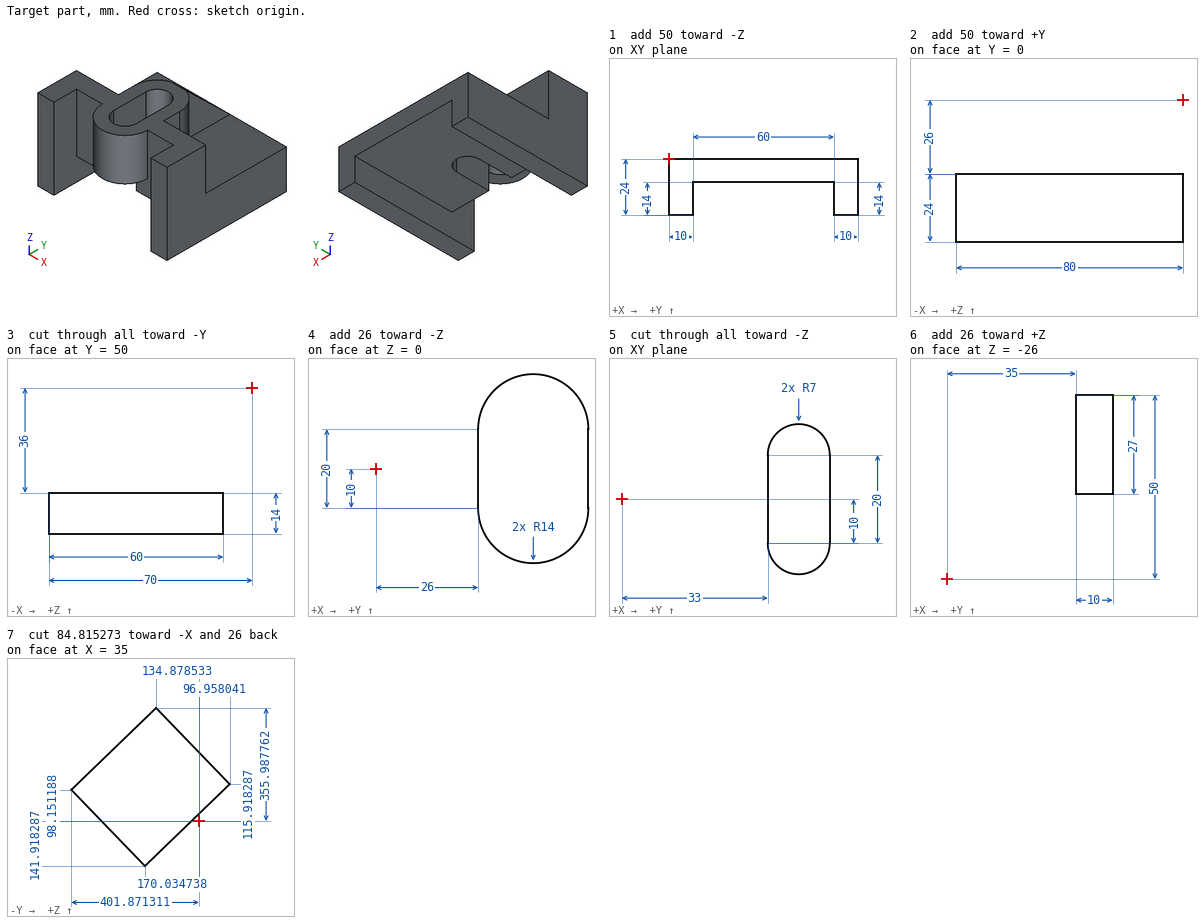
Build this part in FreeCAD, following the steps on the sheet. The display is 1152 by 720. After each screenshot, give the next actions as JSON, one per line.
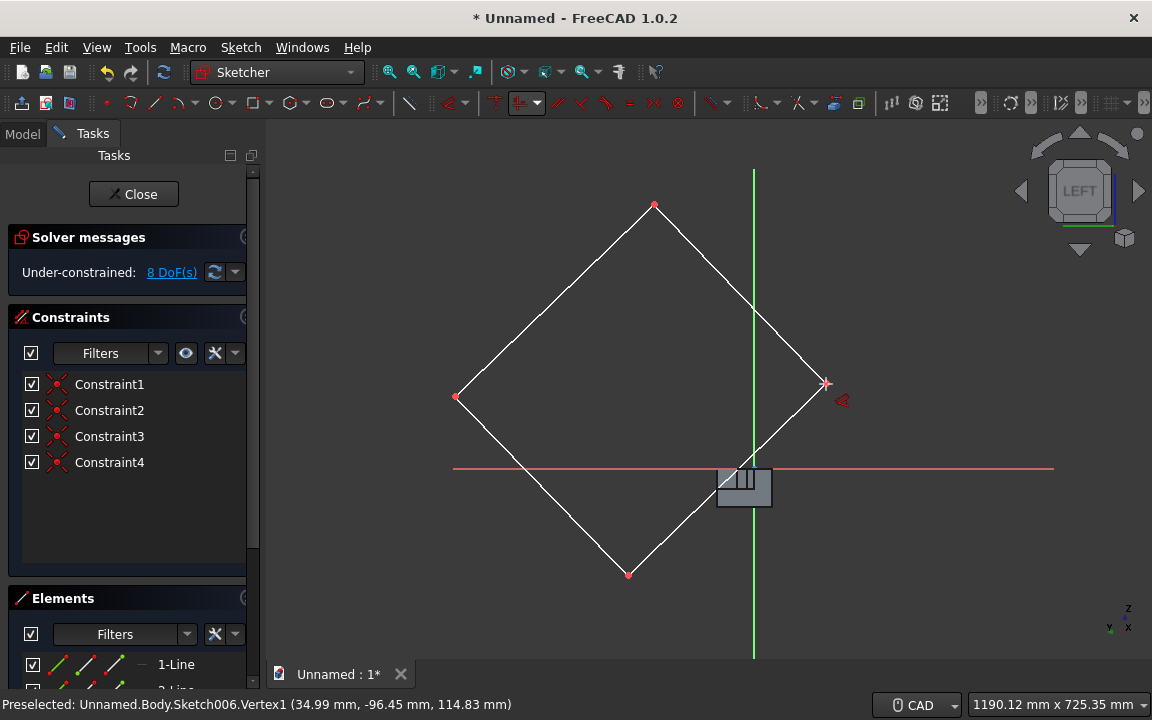
{"action": "left_click", "coordinate": [826, 384]}
{"action": "left_click", "coordinate": [790, 503]}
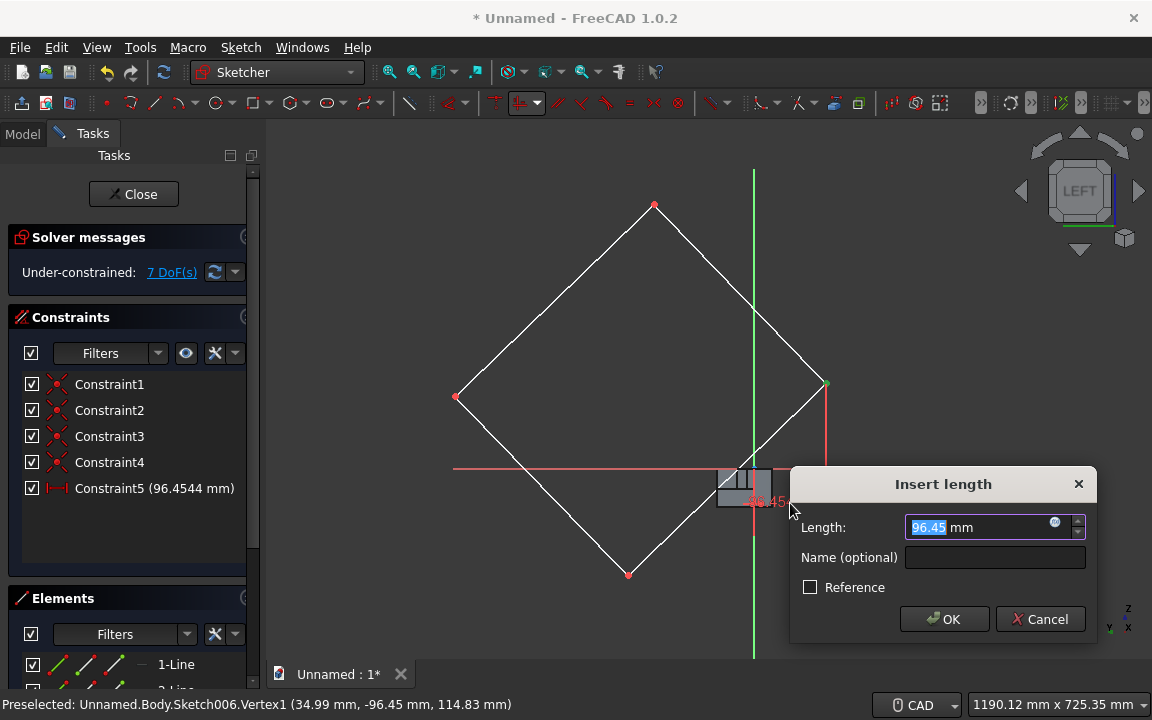
{"action": "type", "text": "96.958041"}
{"action": "key", "text": "Return"}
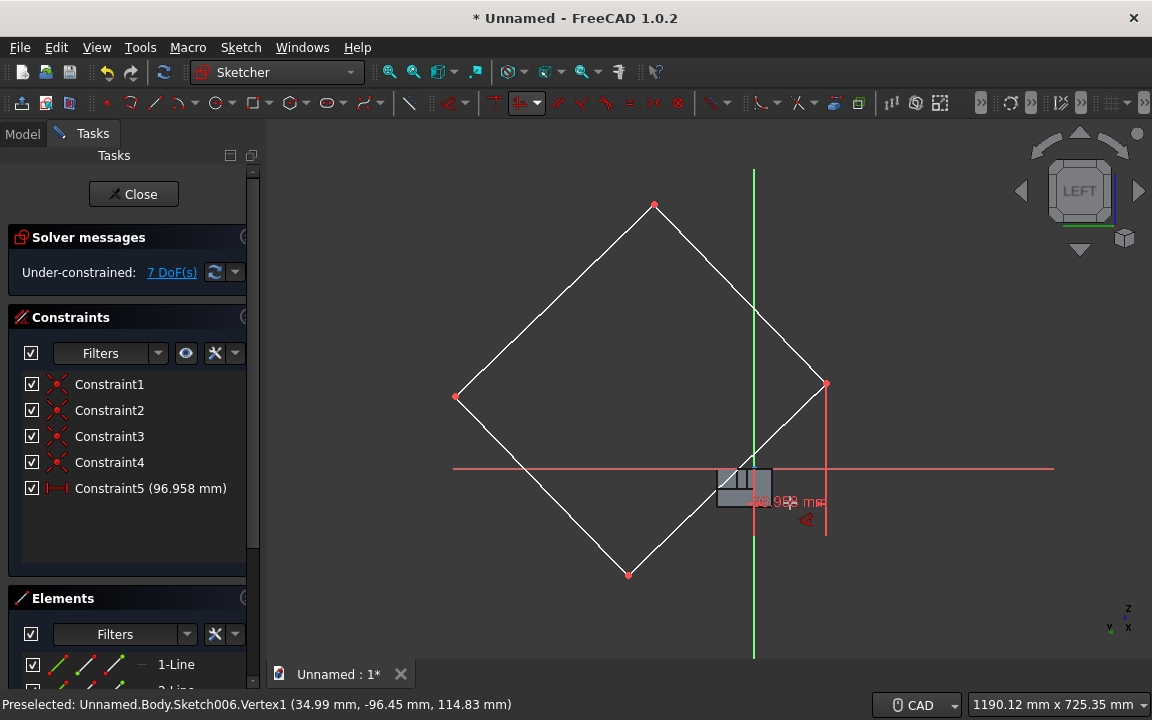
{"action": "left_click", "coordinate": [455, 397]}
{"action": "left_click", "coordinate": [421, 433]}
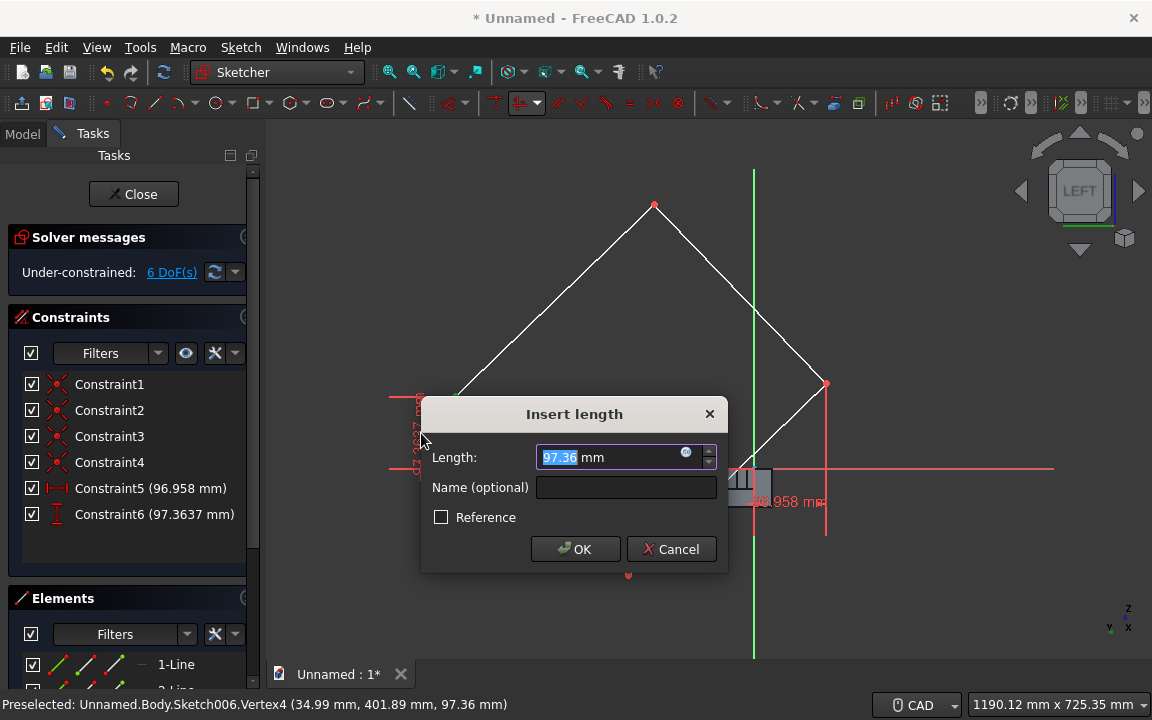
{"action": "type", "text": "98.151188"}
{"action": "key", "text": "Return"}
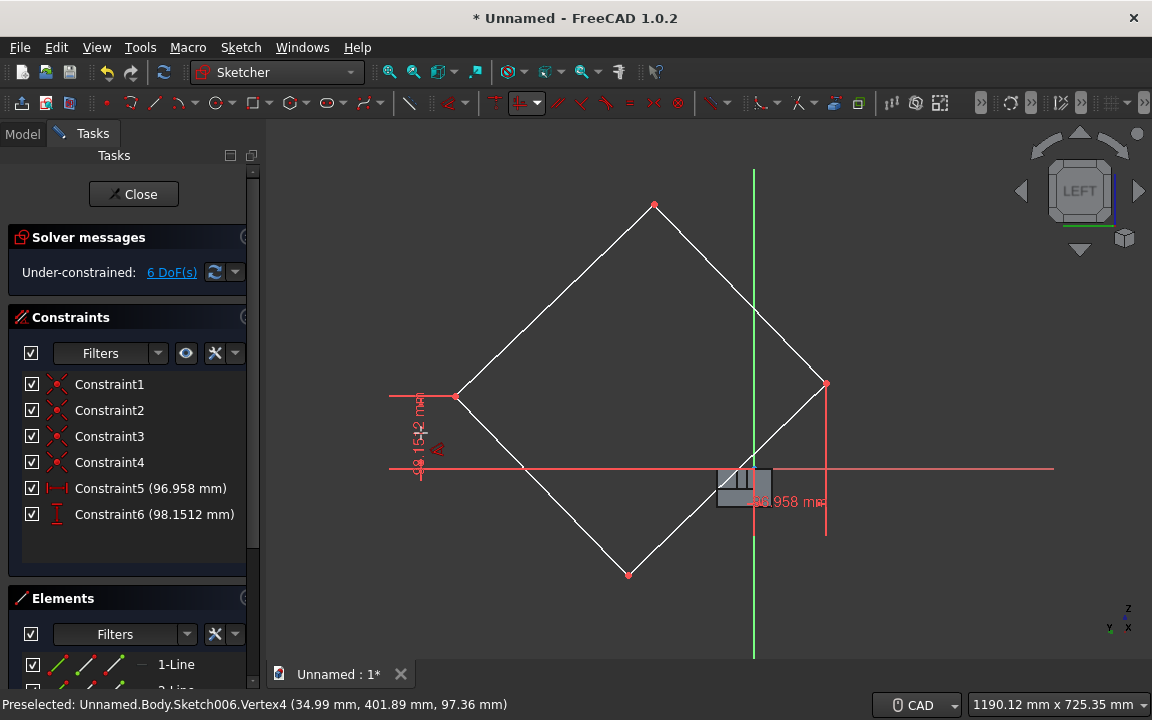
{"action": "left_click", "coordinate": [826, 384]}
{"action": "left_click", "coordinate": [860, 427]}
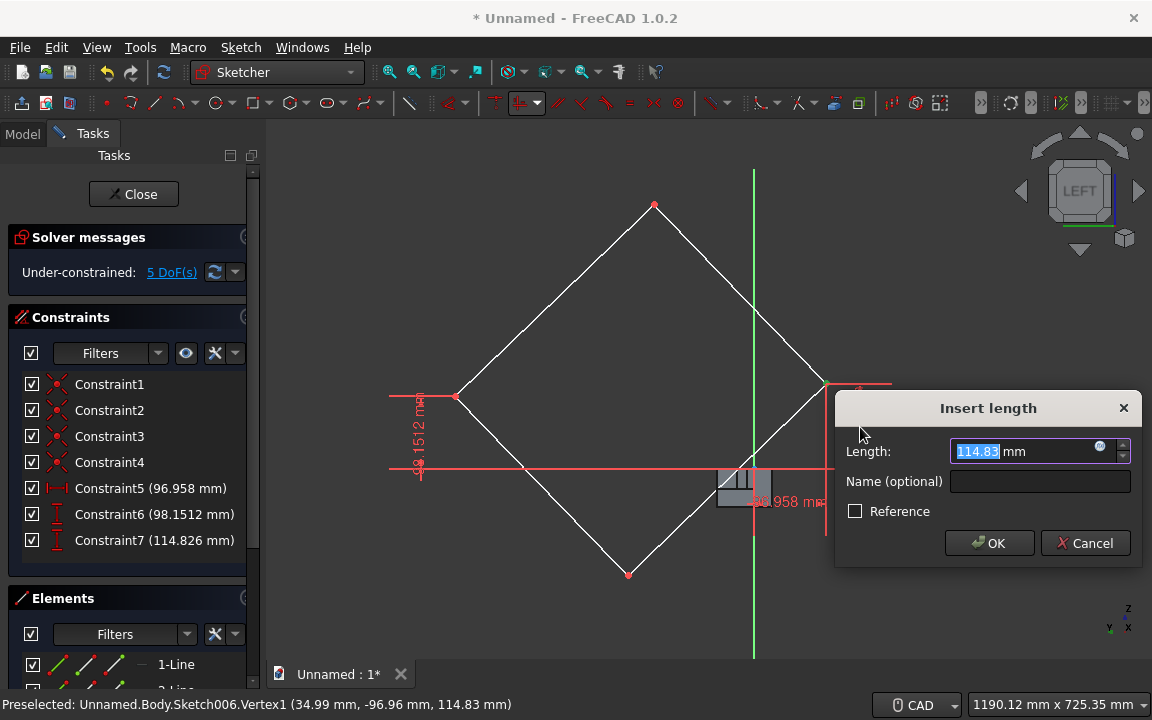
{"action": "type", "text": "115.918287"}
{"action": "key", "text": "Return"}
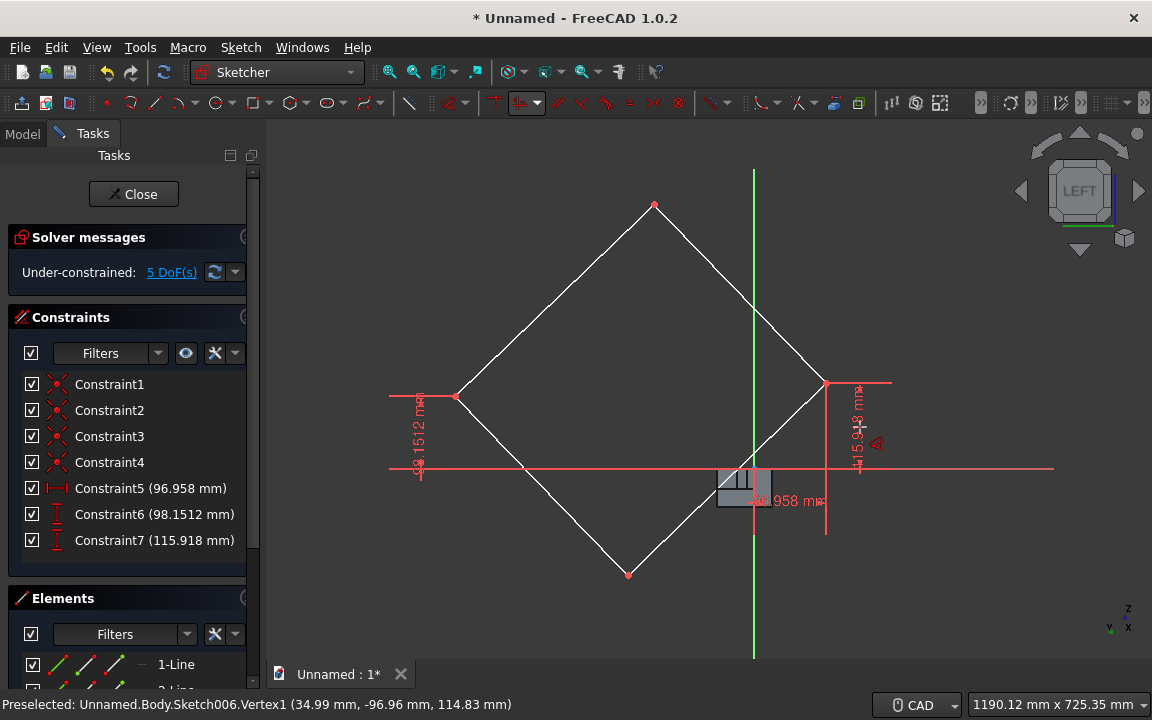
{"action": "left_click", "coordinate": [654, 205]}
{"action": "left_click", "coordinate": [704, 171]}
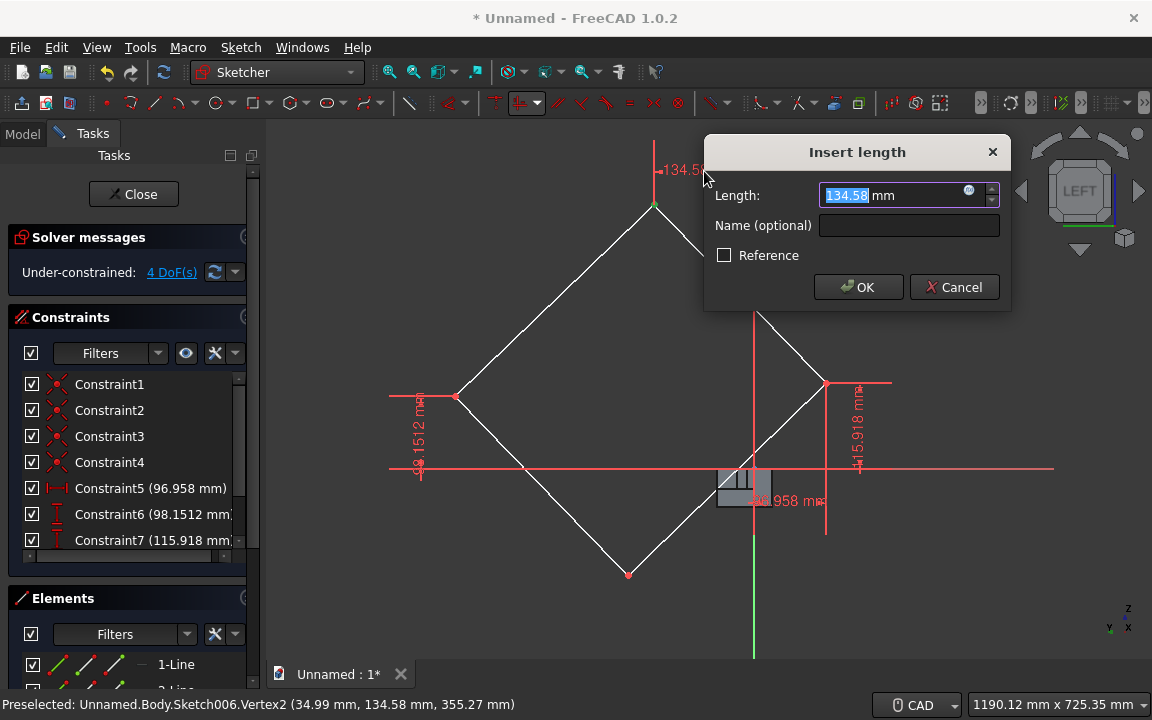
{"action": "type", "text": "134.878533"}
{"action": "key", "text": "Return"}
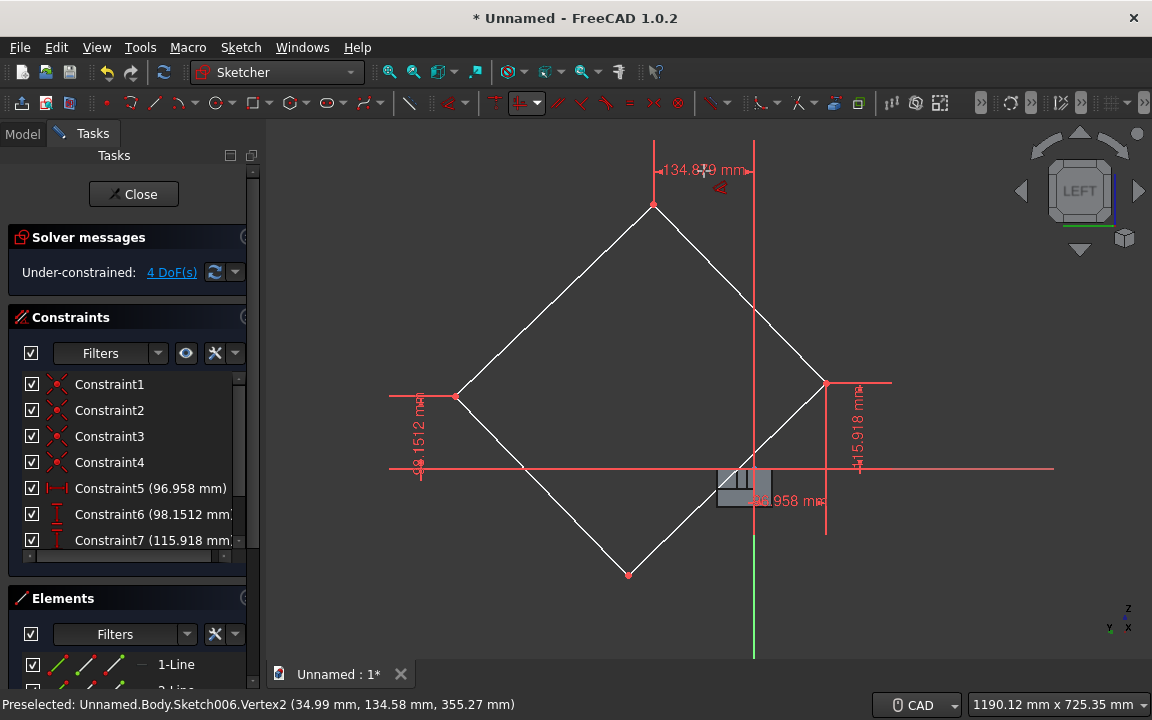
{"action": "left_click", "coordinate": [654, 205]}
{"action": "left_click", "coordinate": [788, 276]}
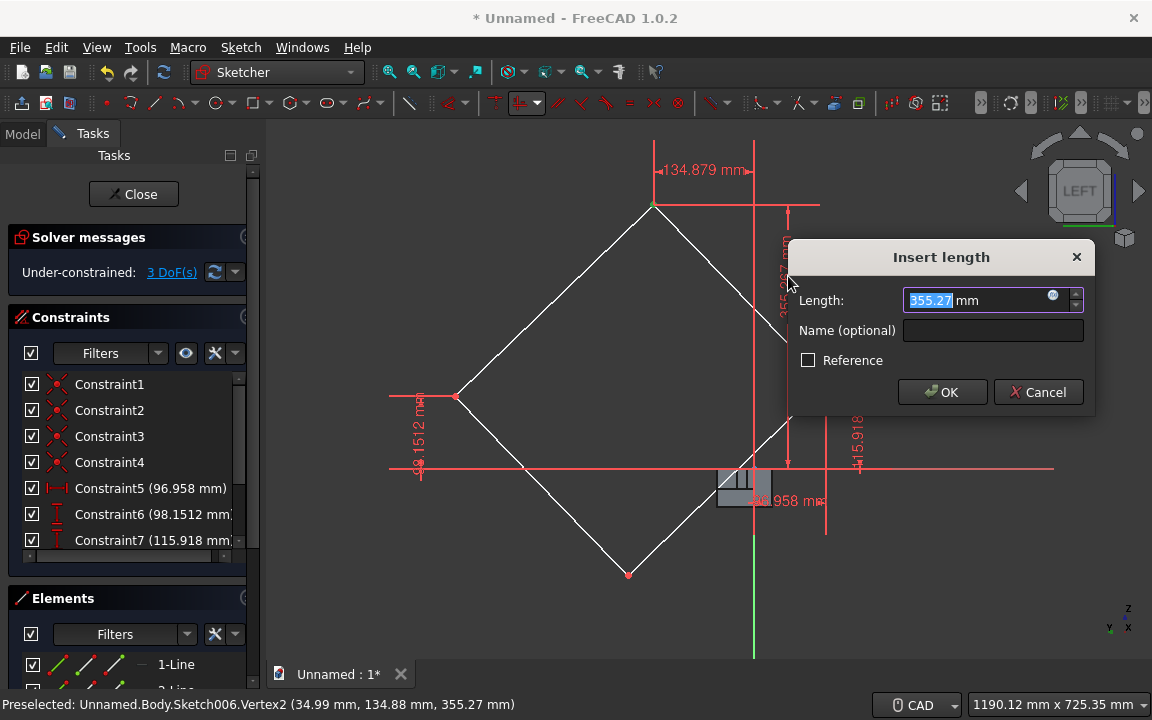
{"action": "type", "text": "355.987762"}
{"action": "key", "text": "Return"}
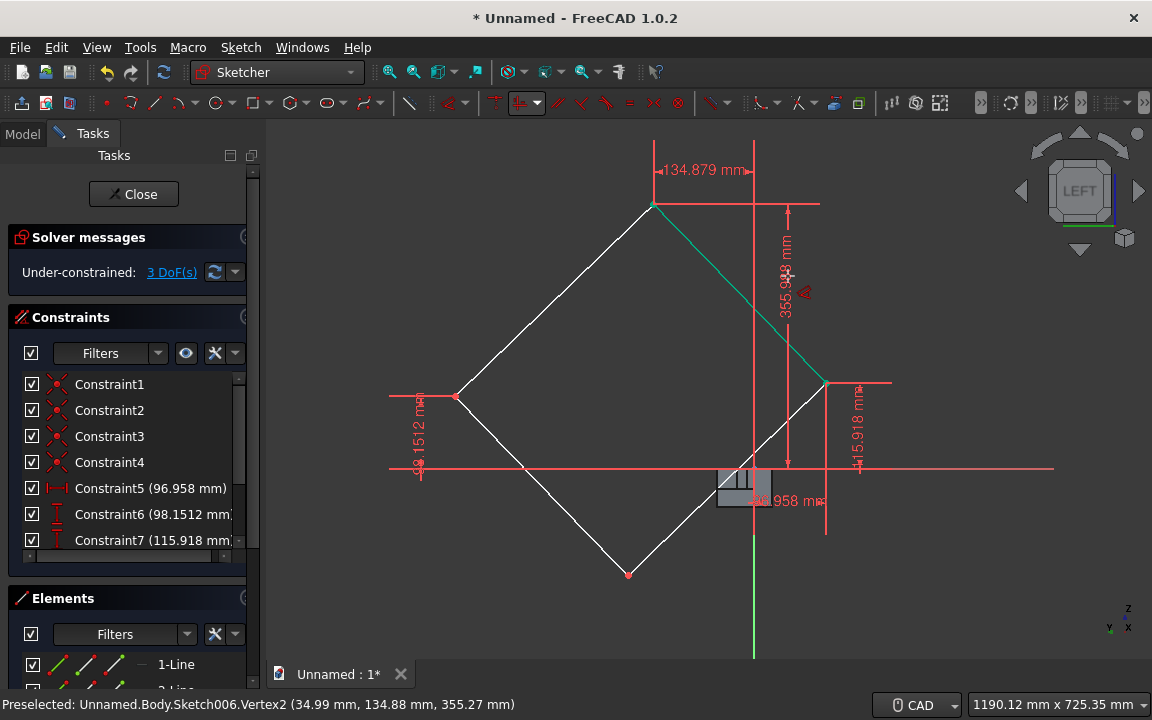
{"action": "left_click", "coordinate": [455, 396]}
{"action": "left_click", "coordinate": [605, 503]}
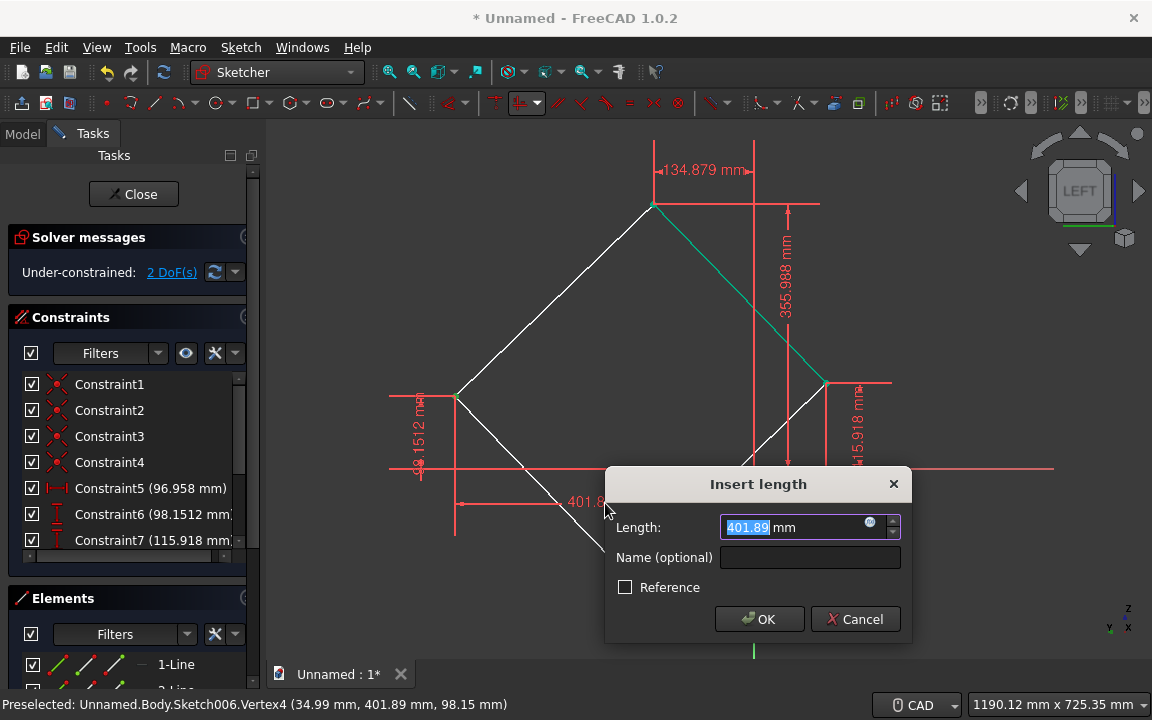
{"action": "type", "text": "401.871311"}
{"action": "key", "text": "Return"}